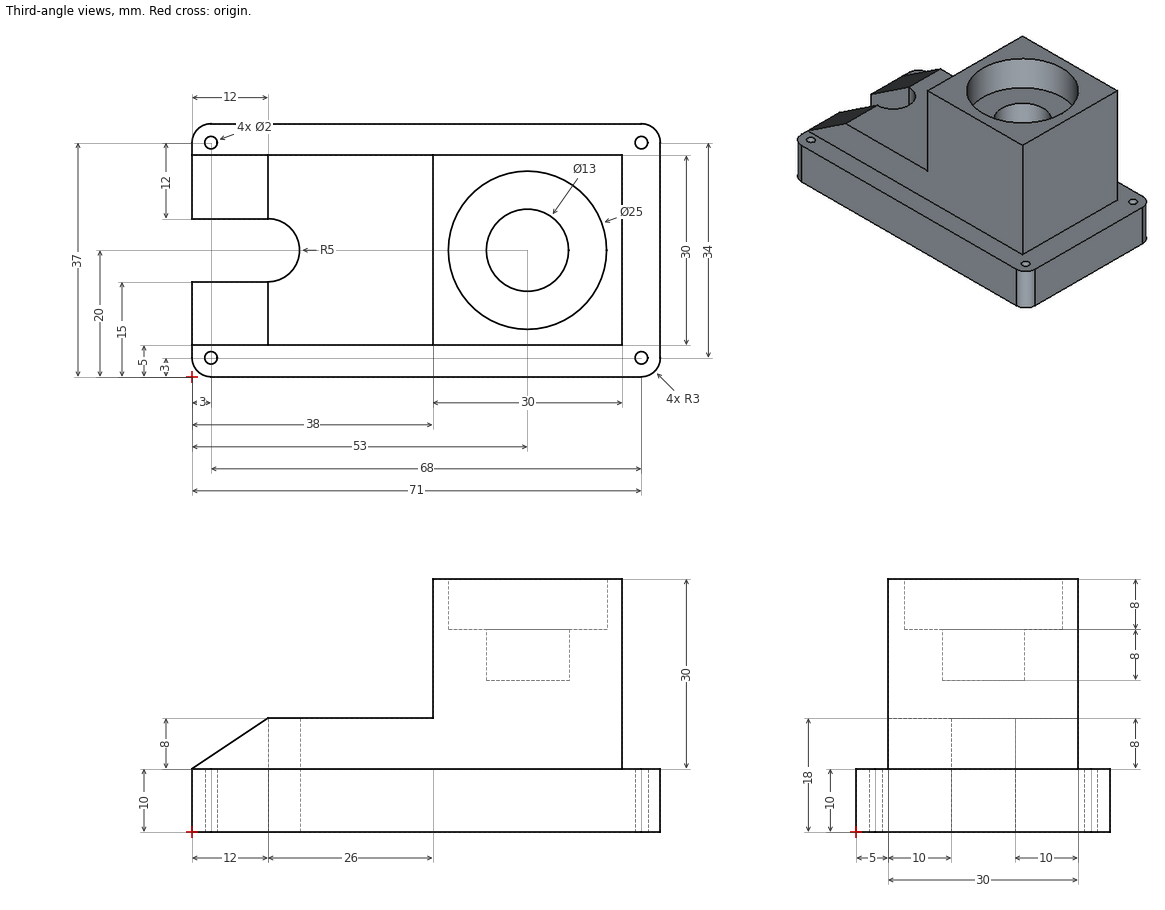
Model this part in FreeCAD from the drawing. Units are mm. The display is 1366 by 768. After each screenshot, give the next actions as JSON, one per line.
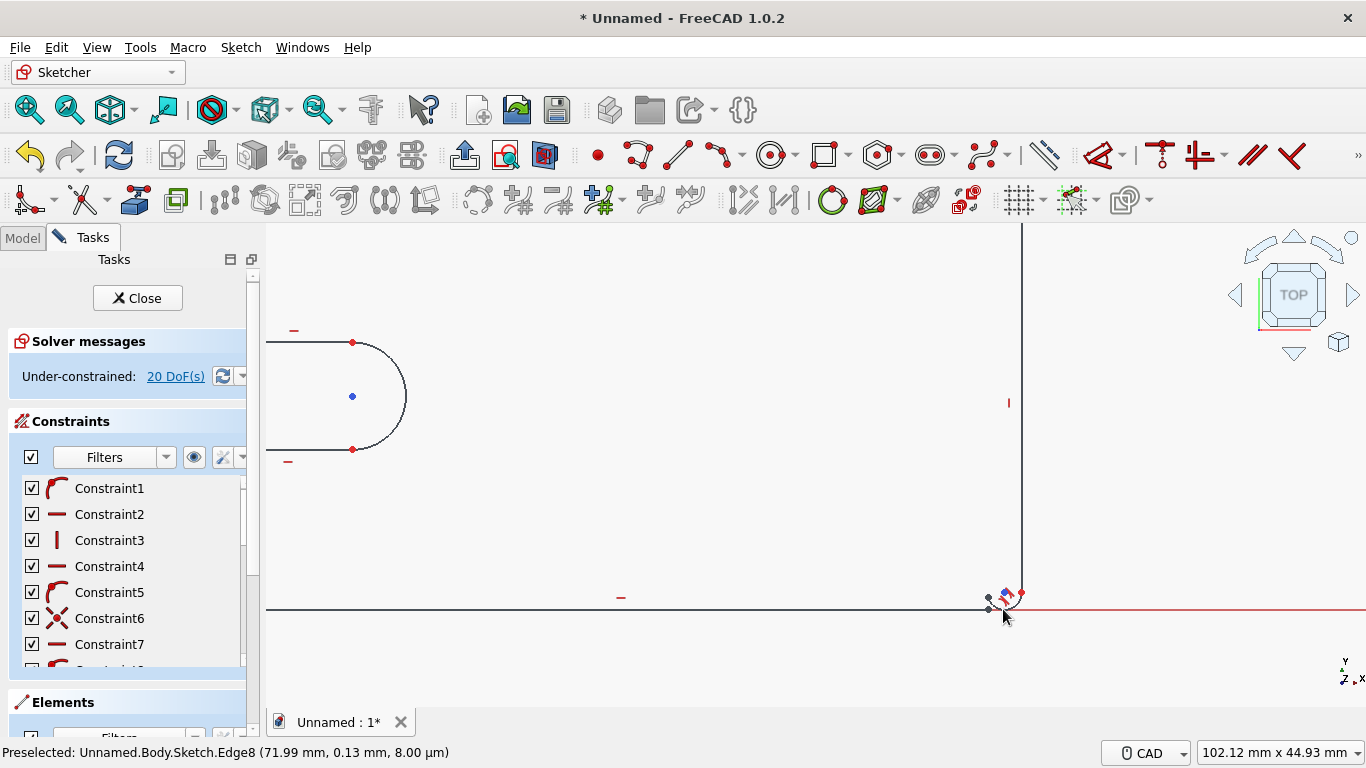
{"action": "left_click", "coordinate": [1022, 479]}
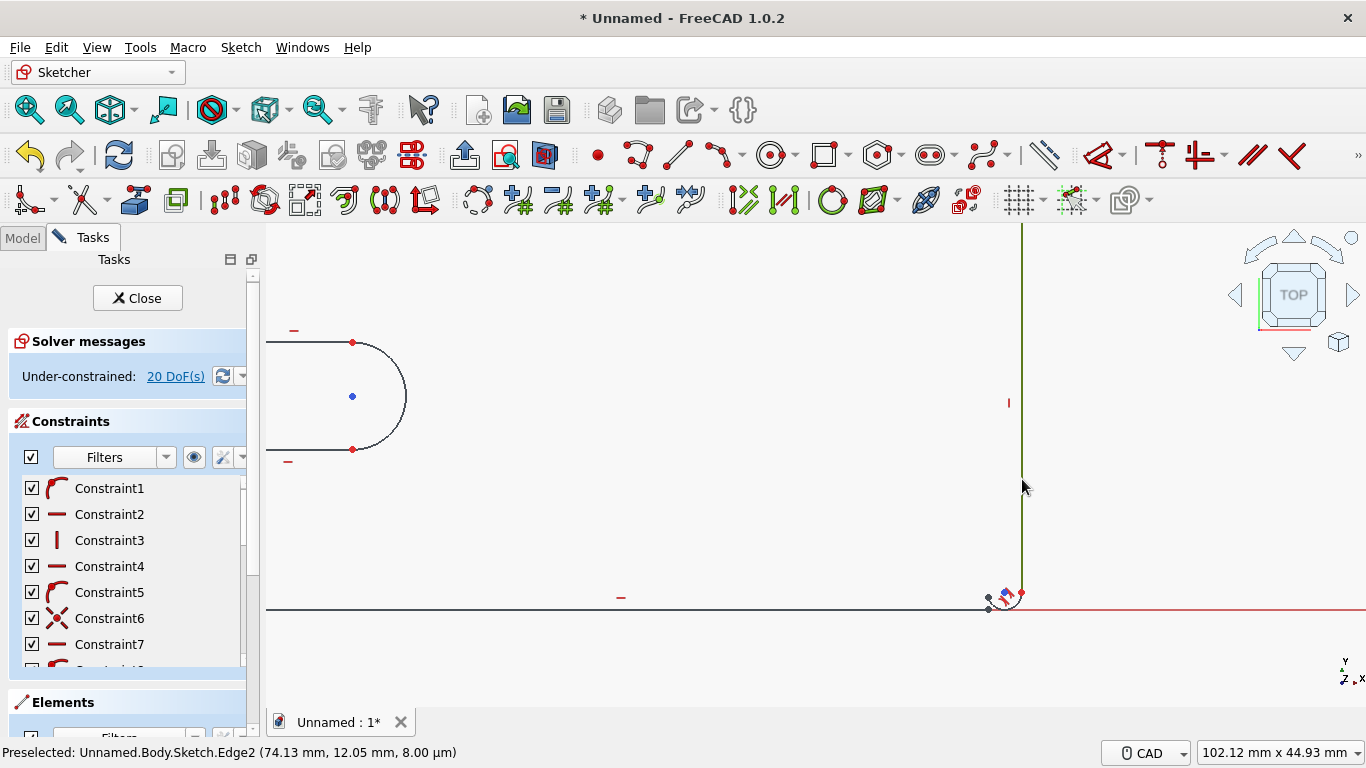
{"action": "scroll", "coordinate": [1003, 609], "scroll_direction": "down", "scroll_amount": 2}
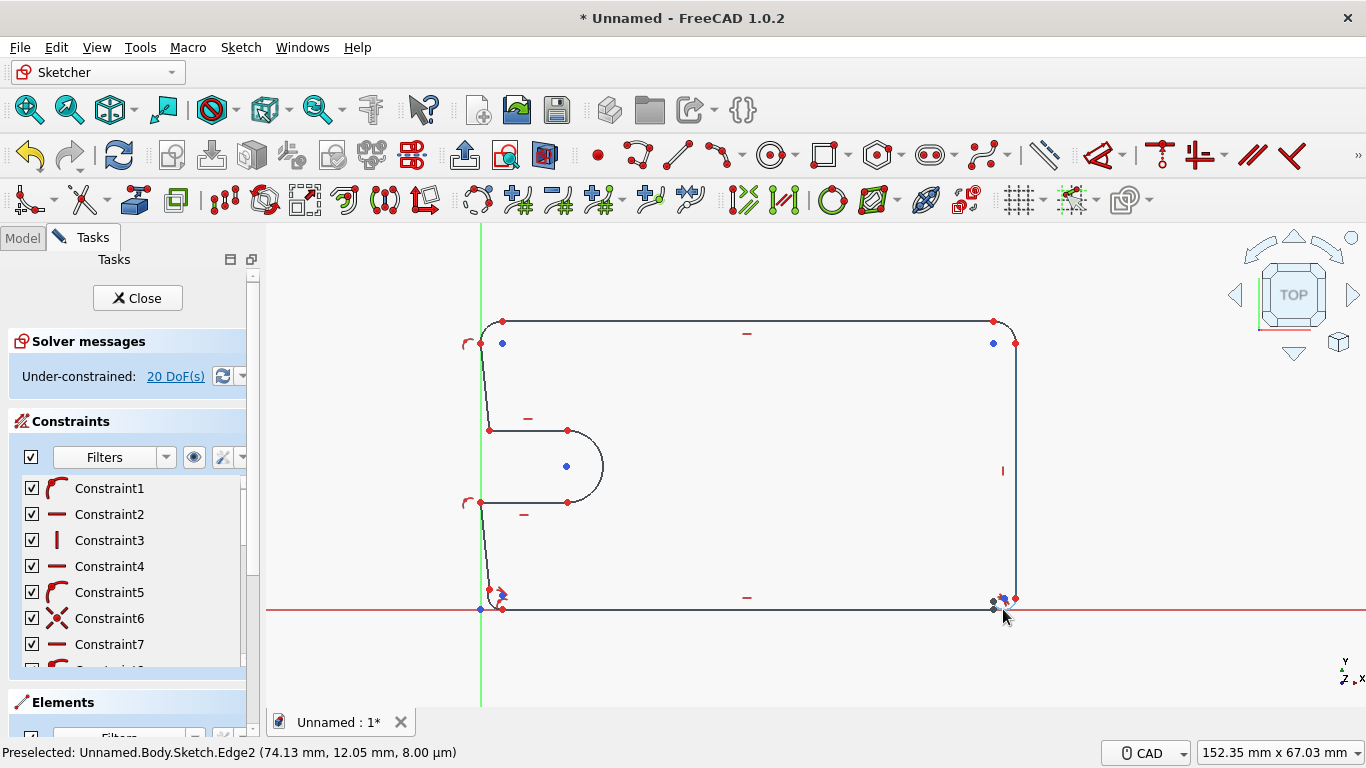
{"action": "scroll", "coordinate": [1013, 333], "scroll_direction": "up", "scroll_amount": 2}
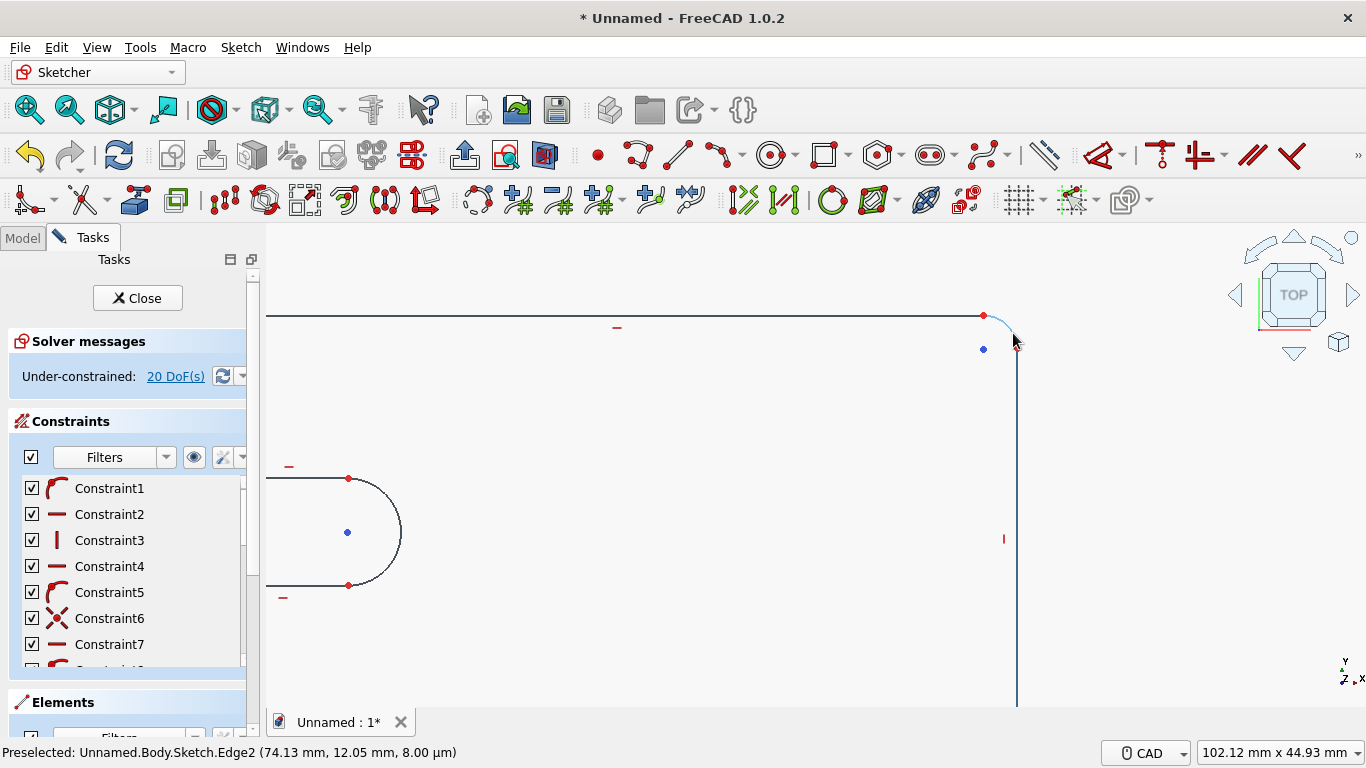
{"action": "left_click", "coordinate": [1013, 334]}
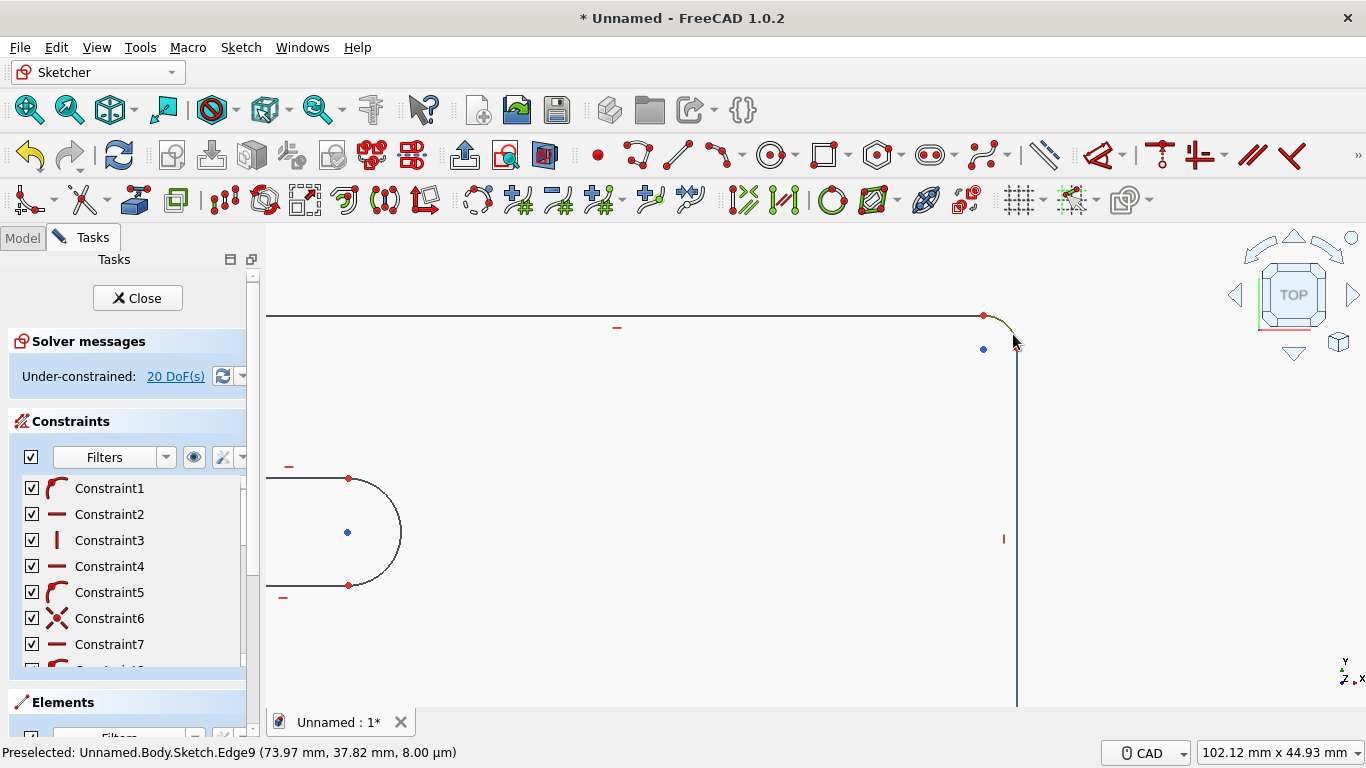
{"action": "key", "text": "t"}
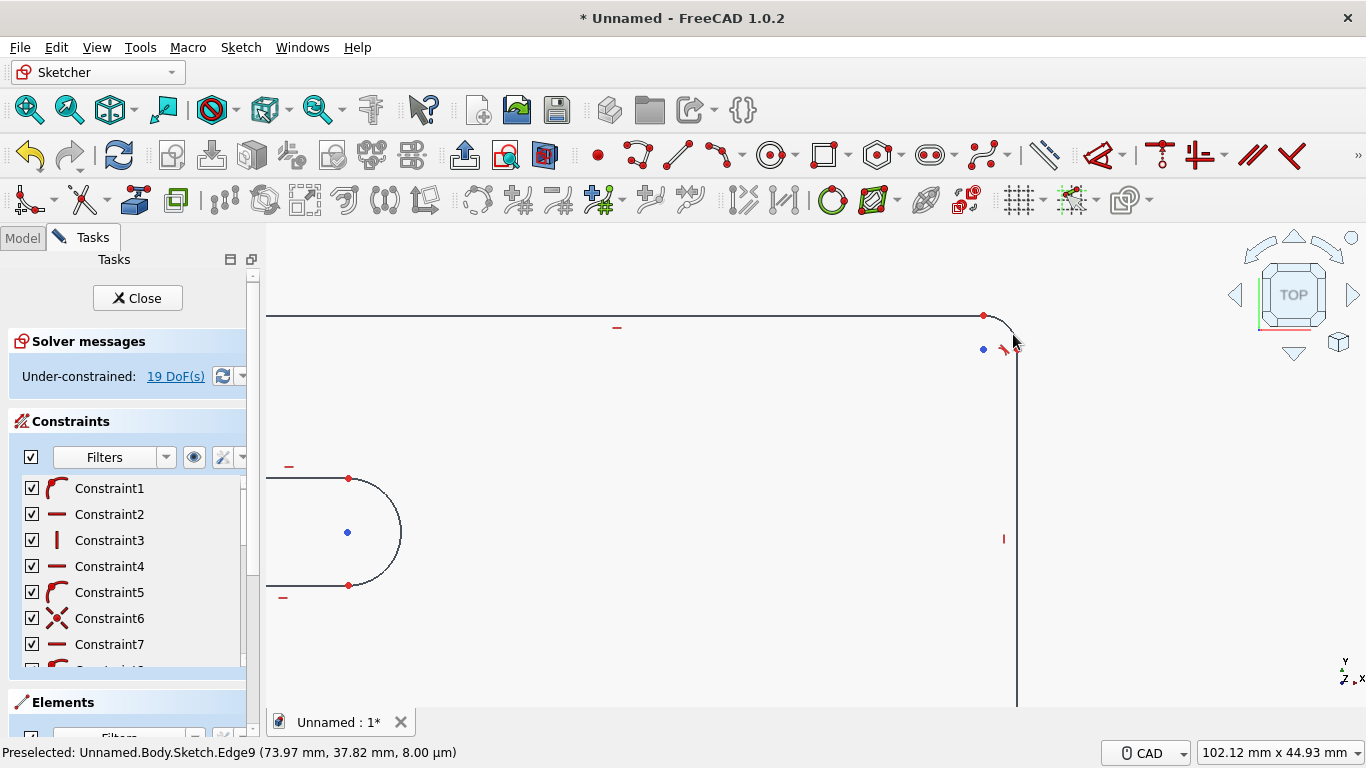
{"action": "left_click", "coordinate": [764, 316]}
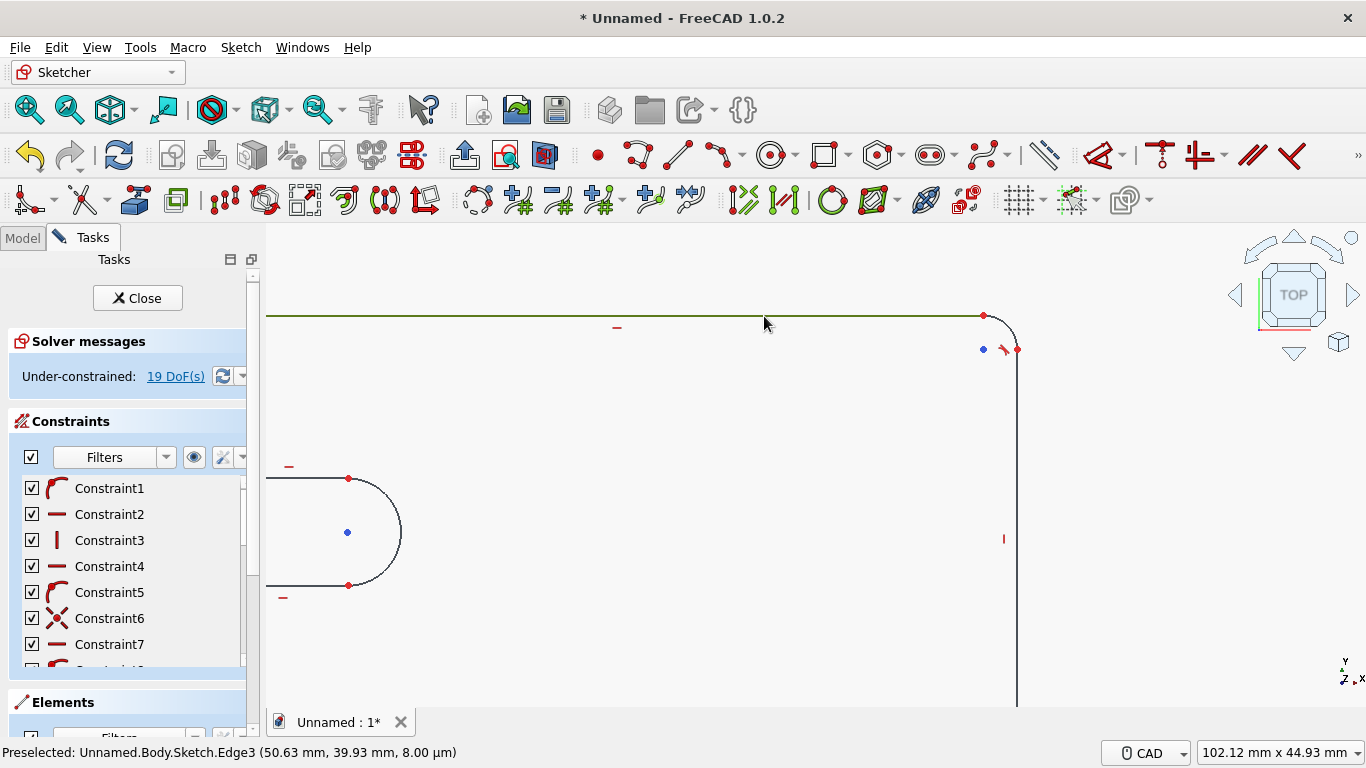
{"action": "left_click", "coordinate": [1013, 334]}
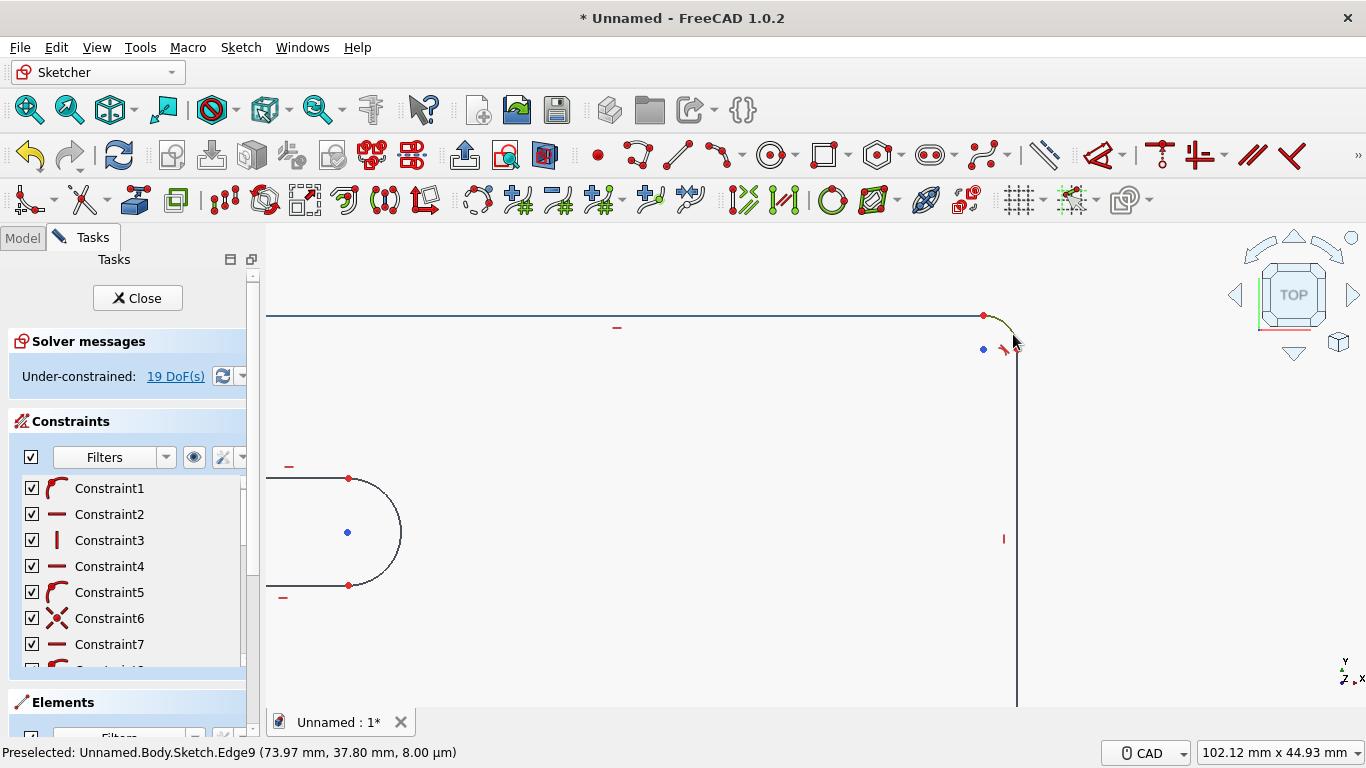
{"action": "key", "text": "t"}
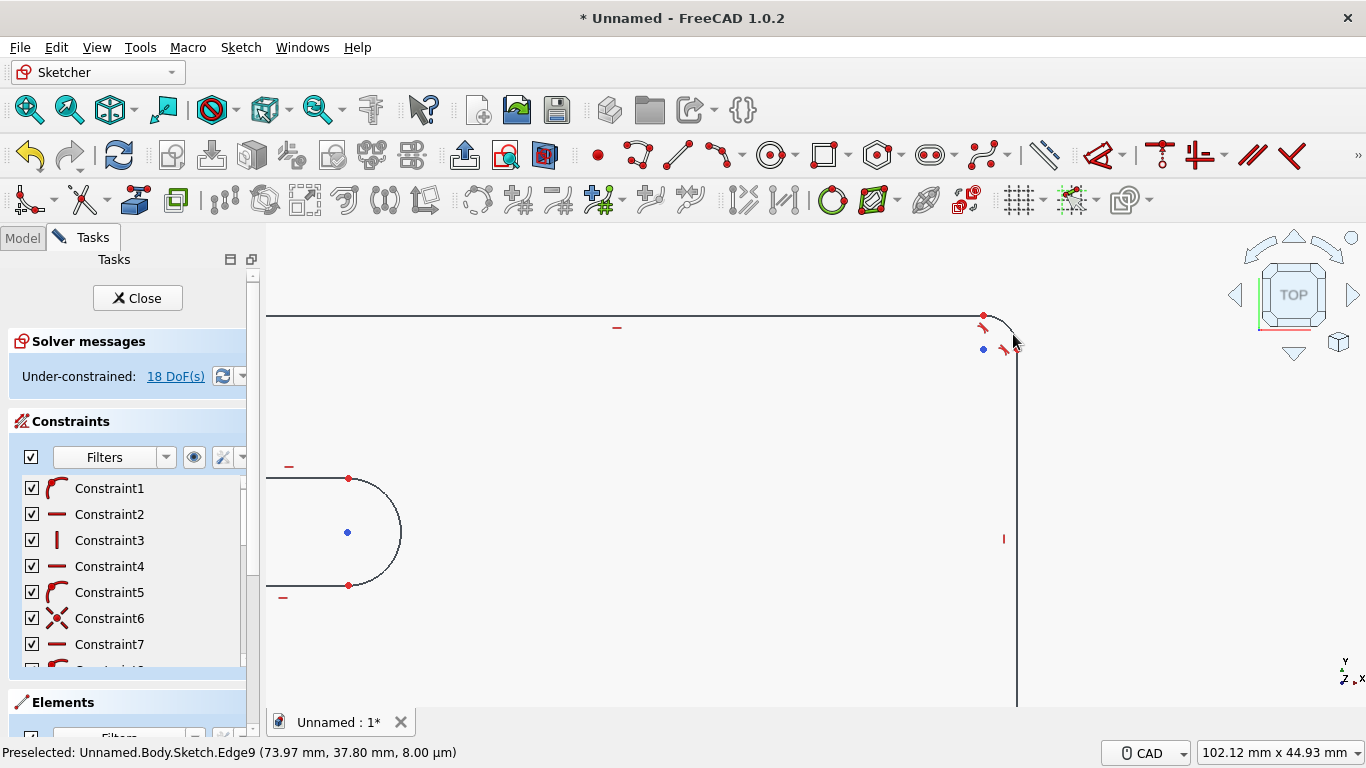
{"action": "left_click", "coordinate": [764, 316]}